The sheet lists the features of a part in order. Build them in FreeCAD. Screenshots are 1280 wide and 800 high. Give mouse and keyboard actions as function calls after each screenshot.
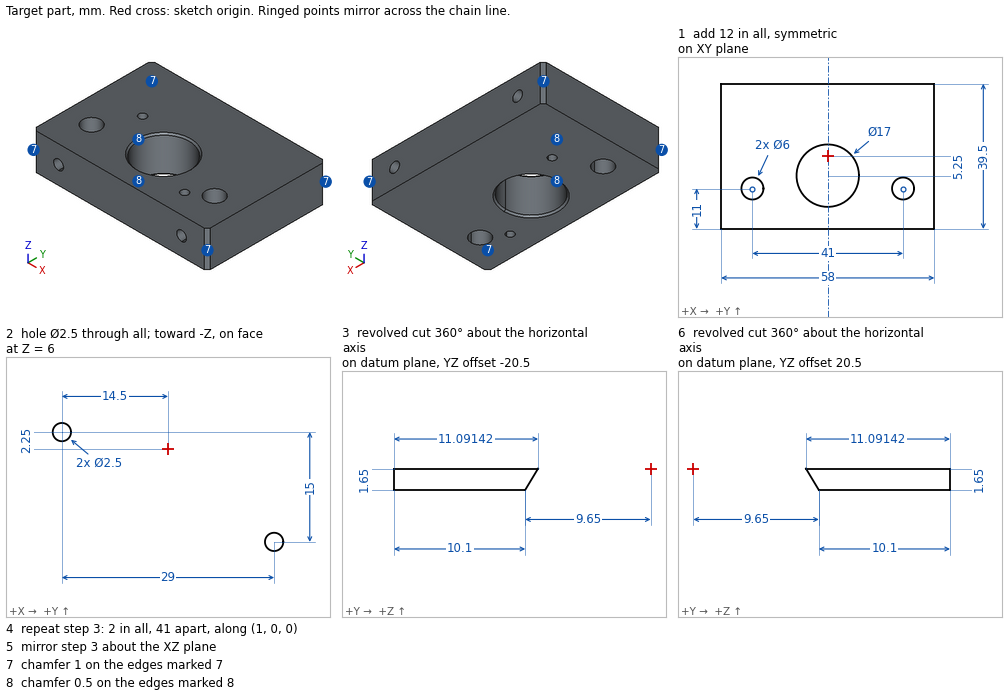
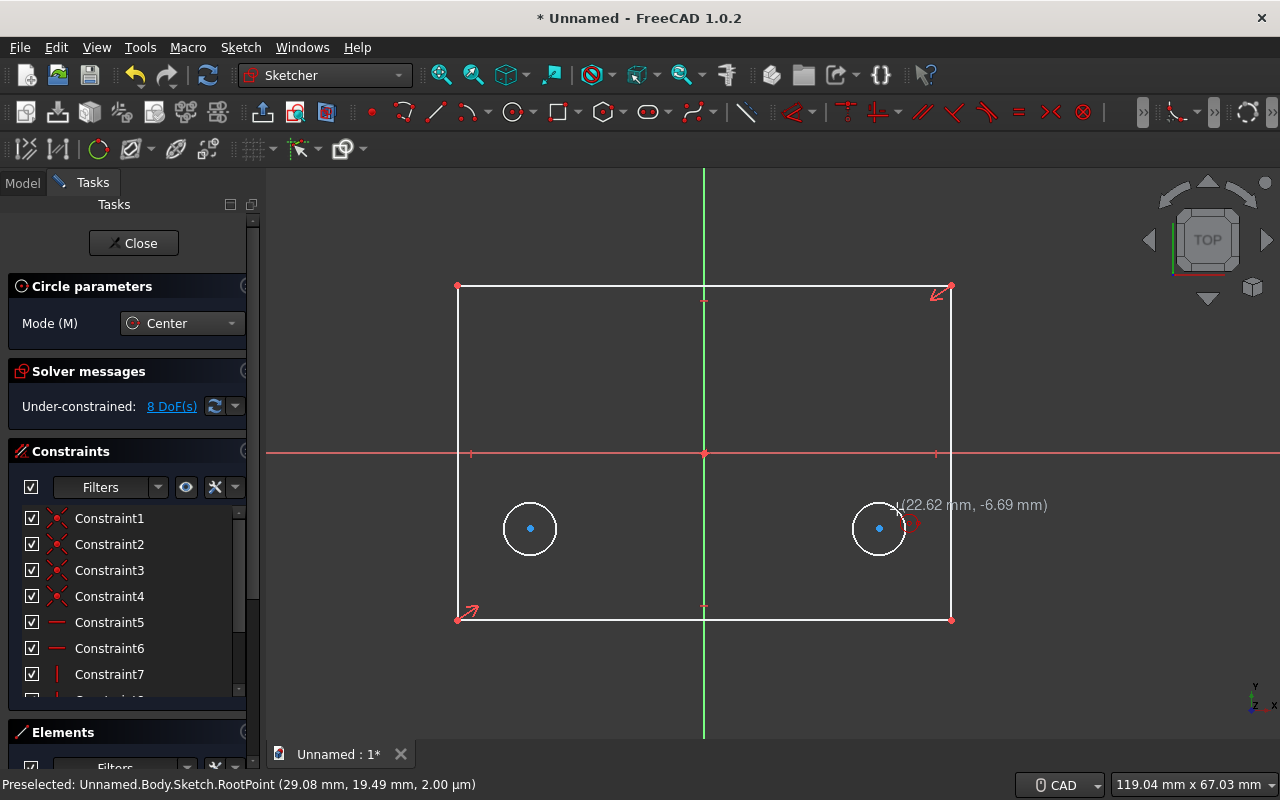
click(704, 498)
click(756, 549)
key(Escape)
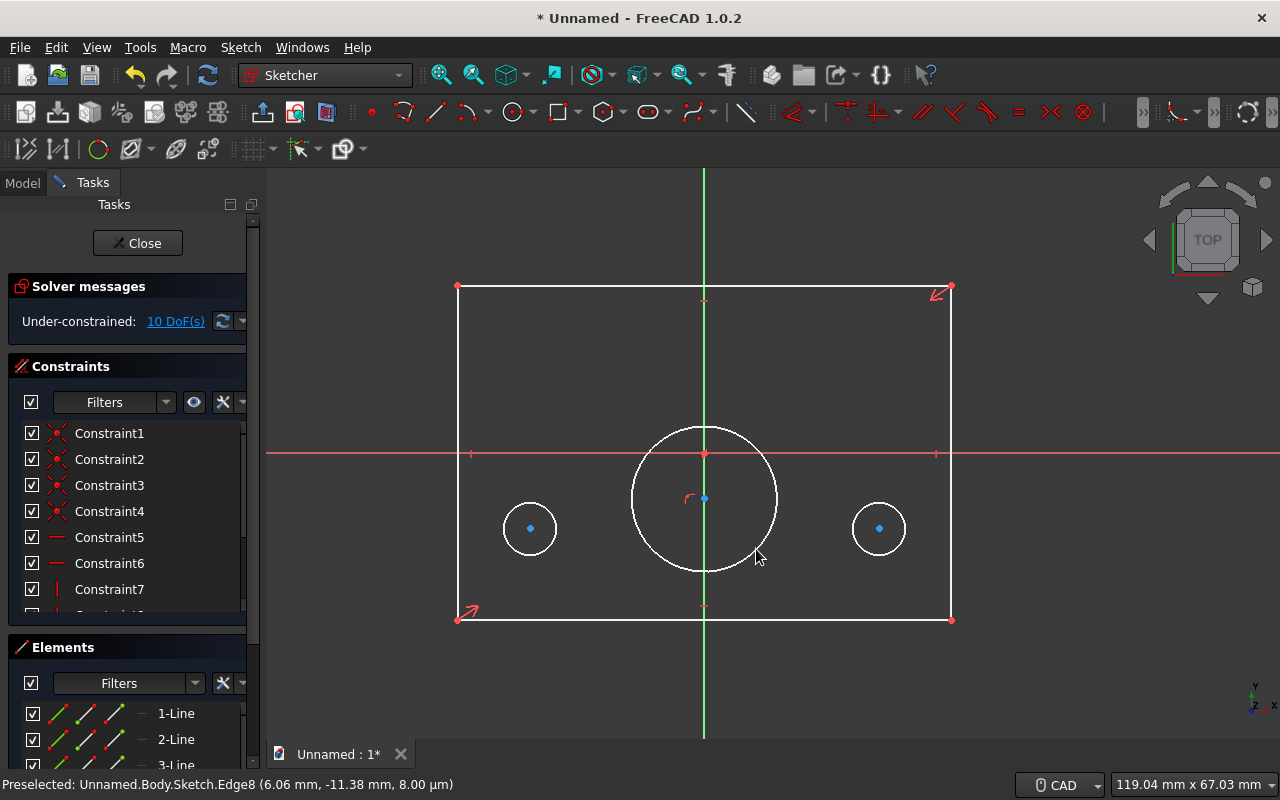
click(548, 510)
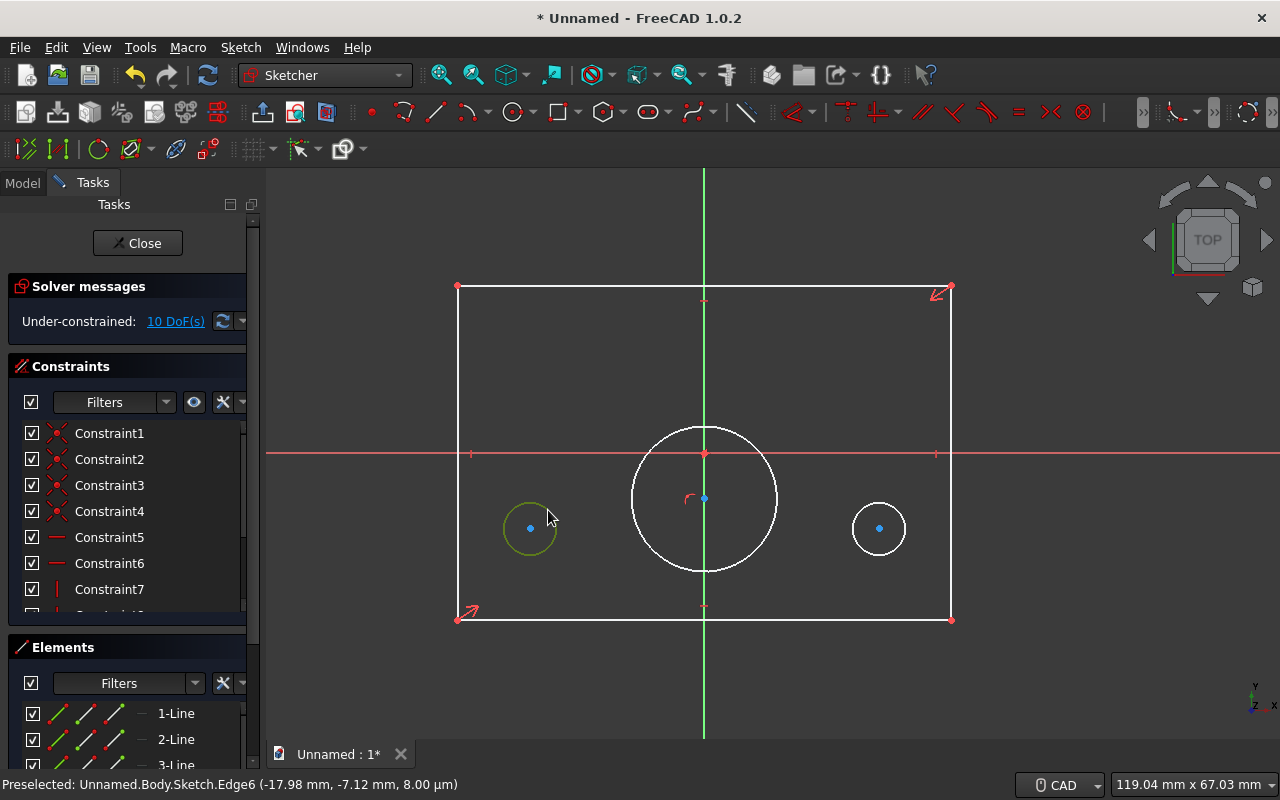
click(897, 510)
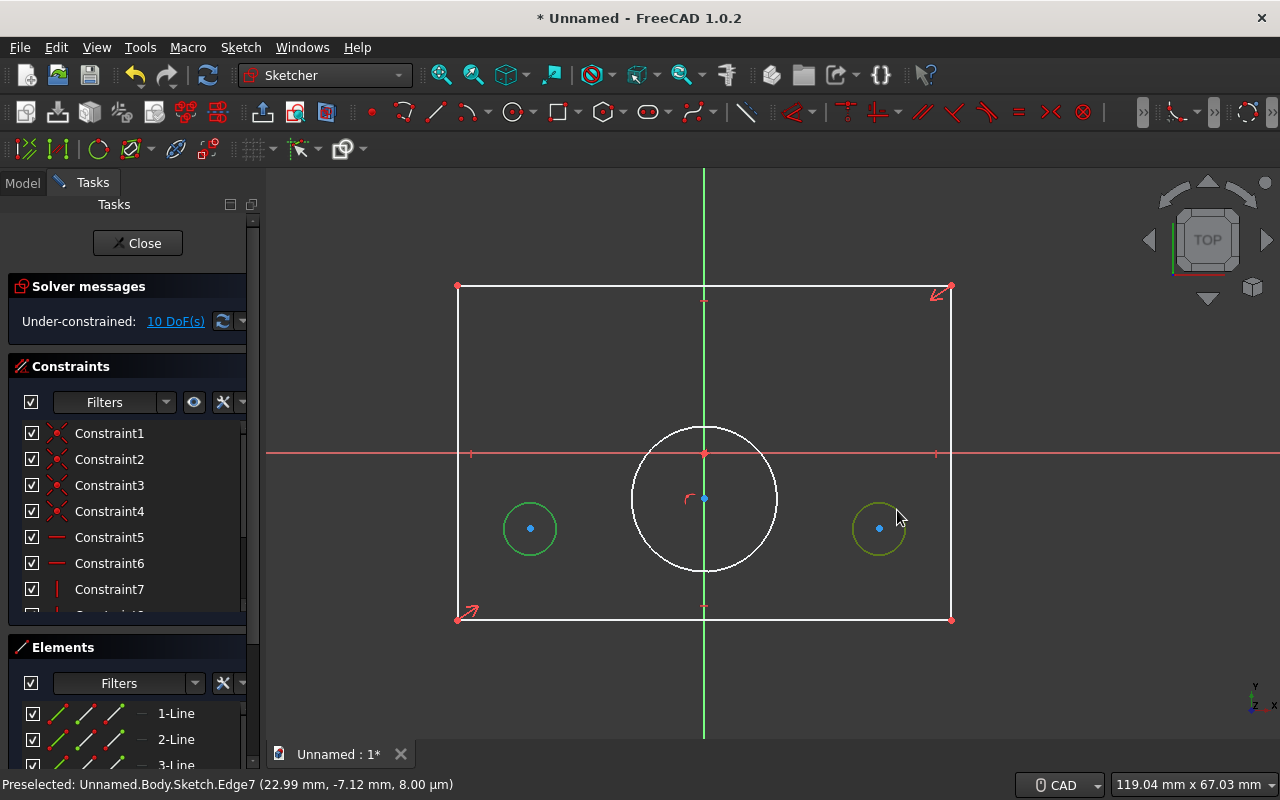
key(e)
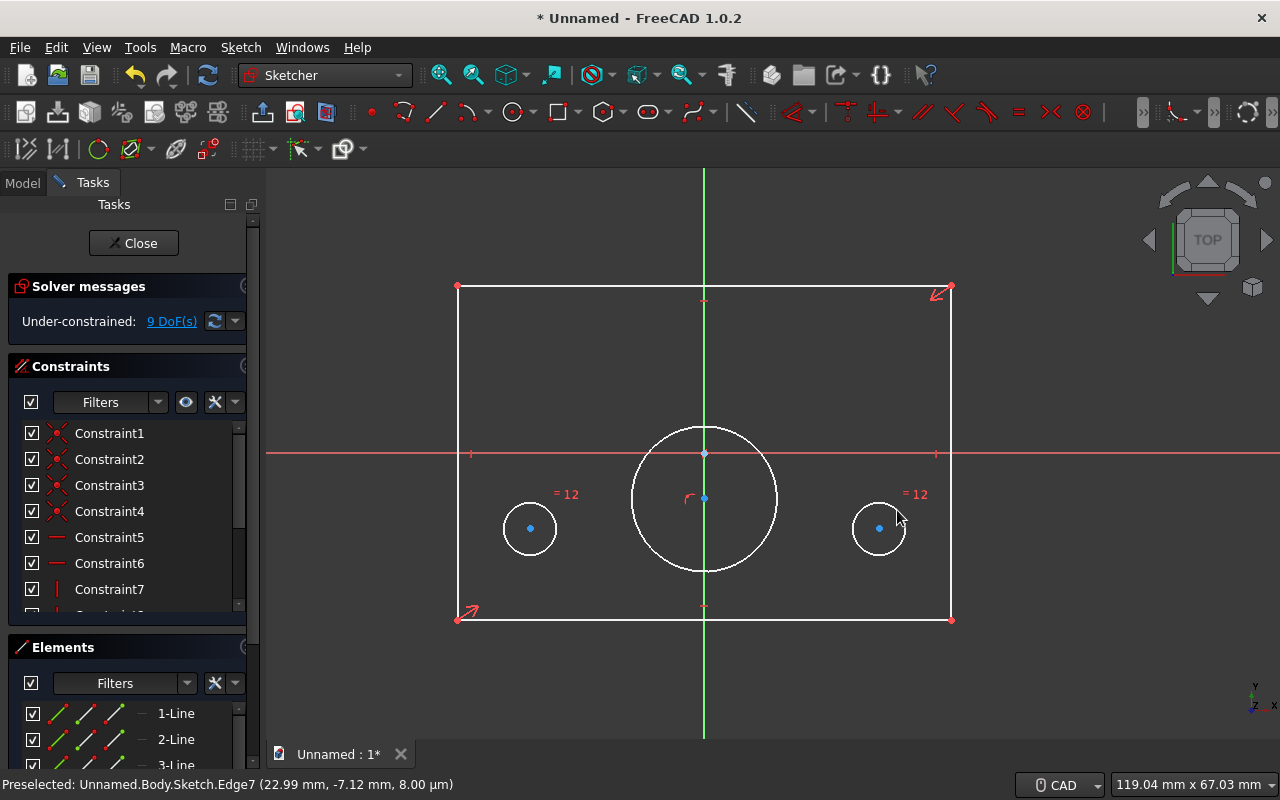
click(530, 529)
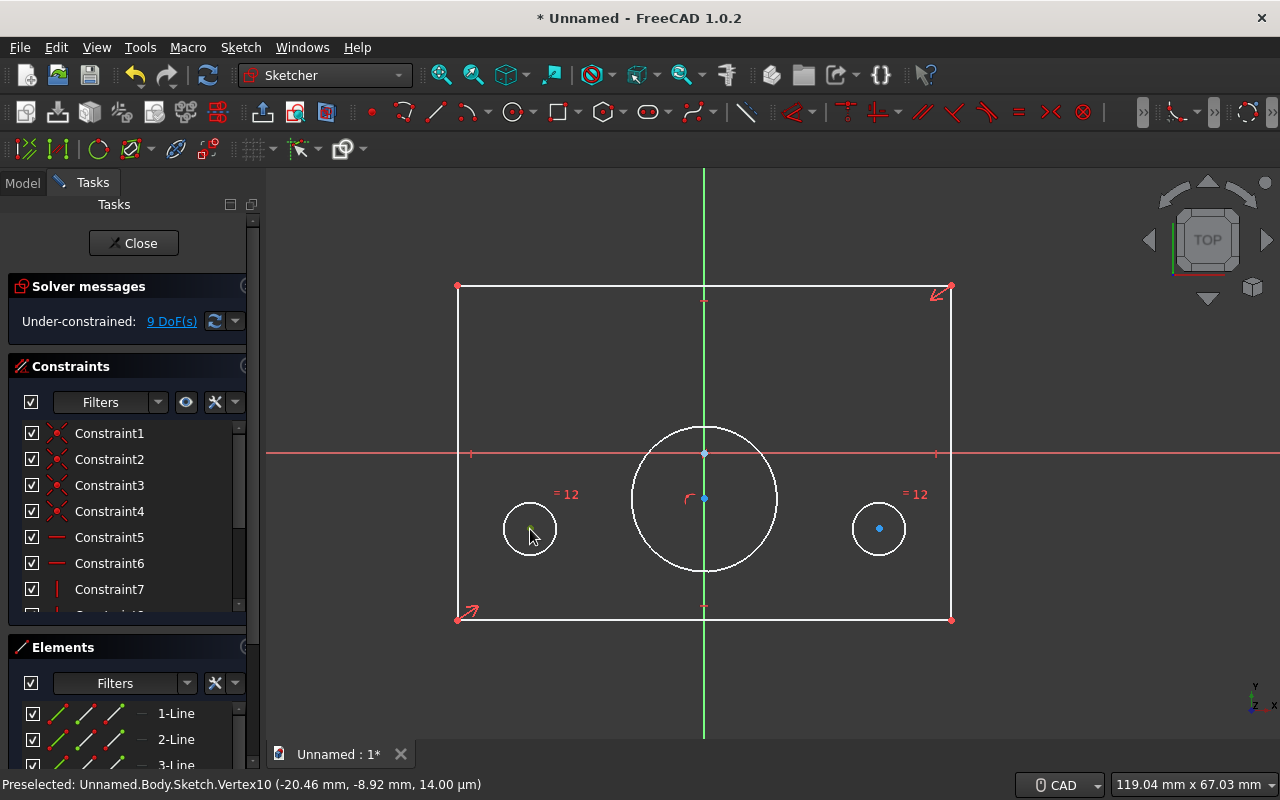
click(879, 529)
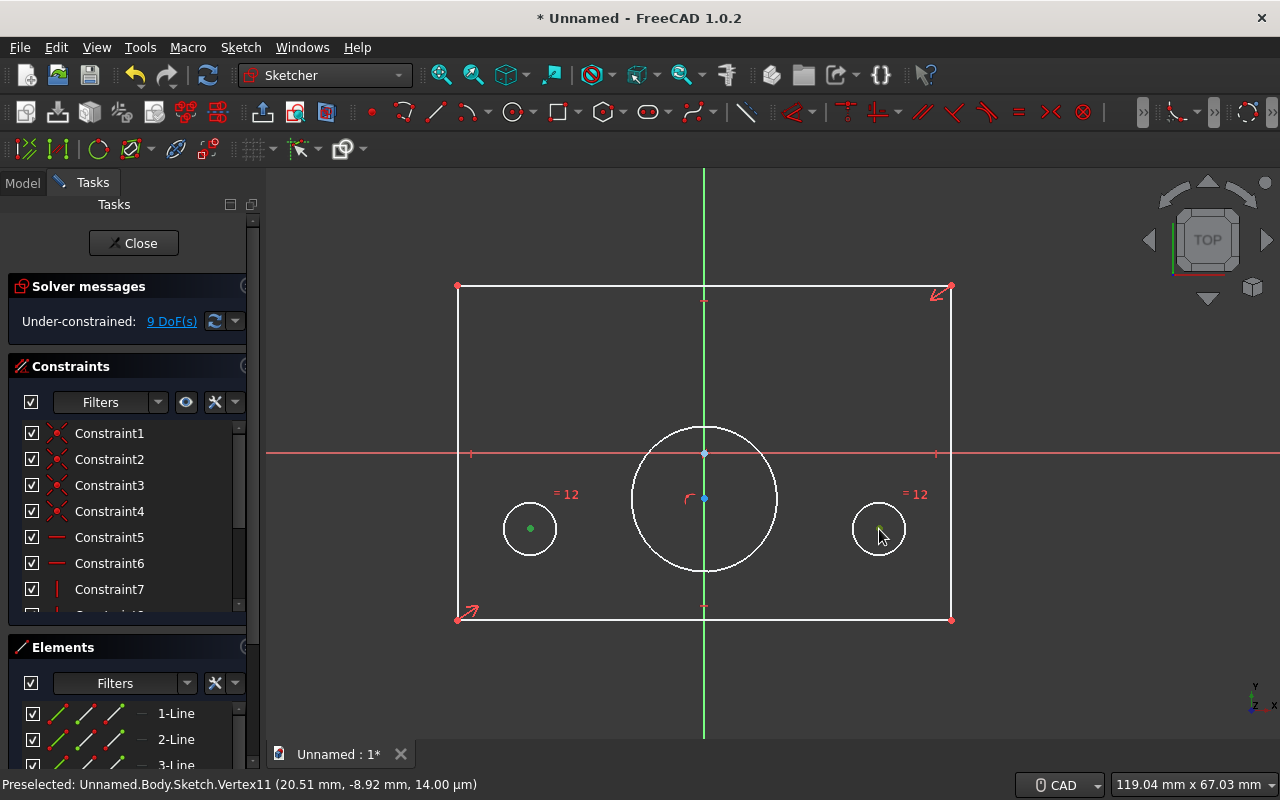
click(704, 674)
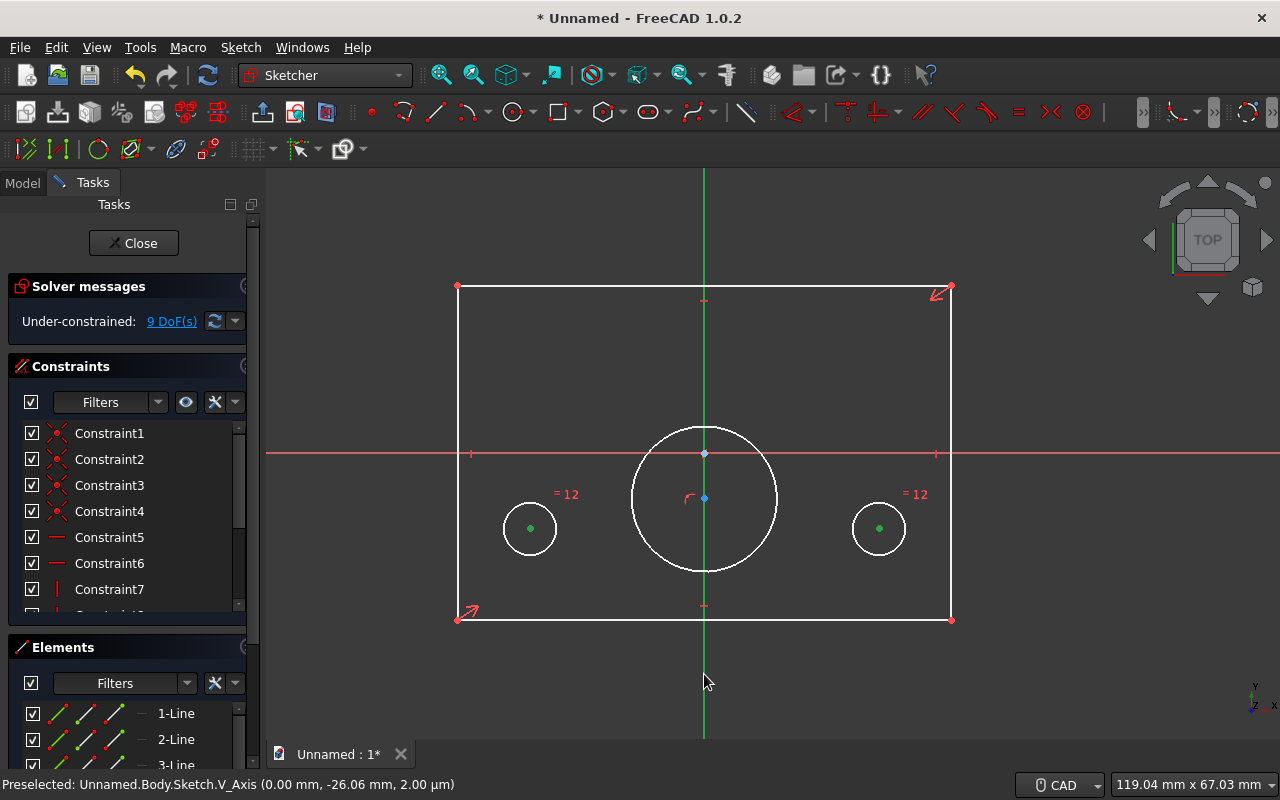
click(1052, 112)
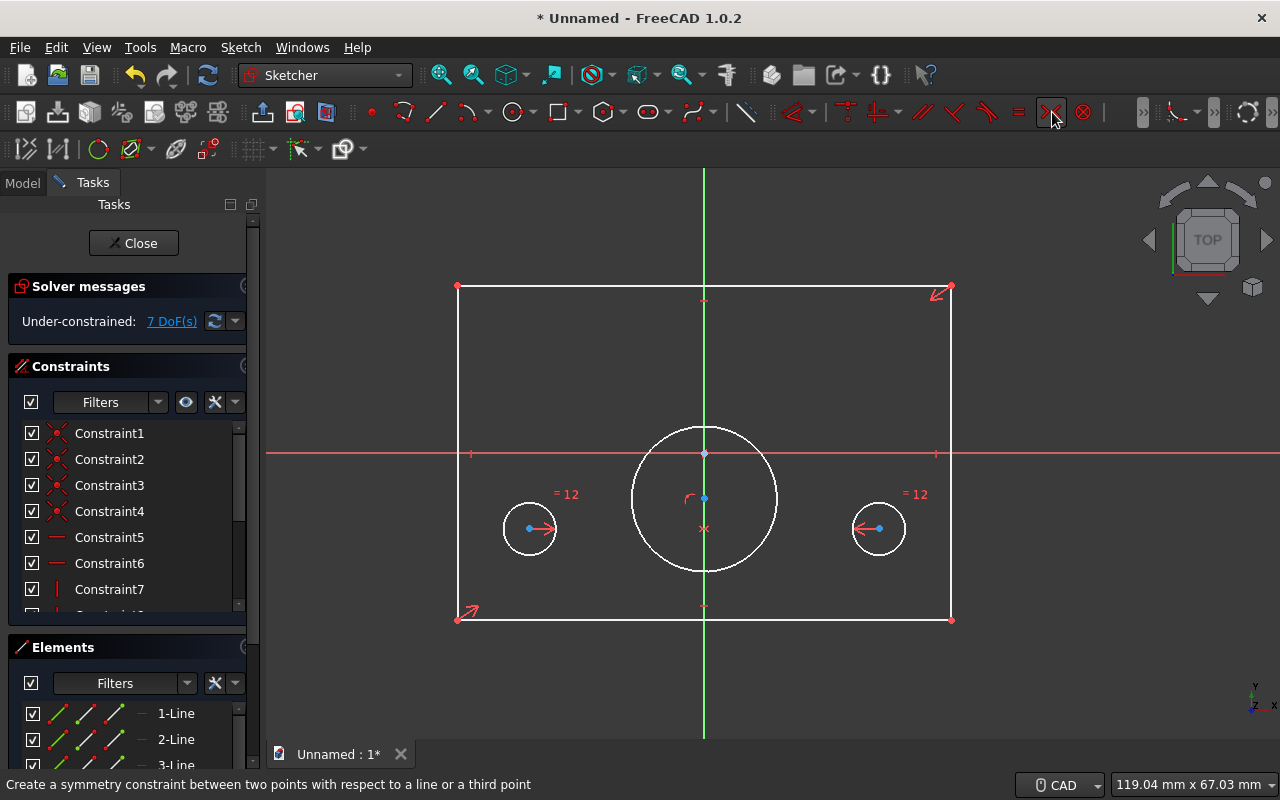
key(d)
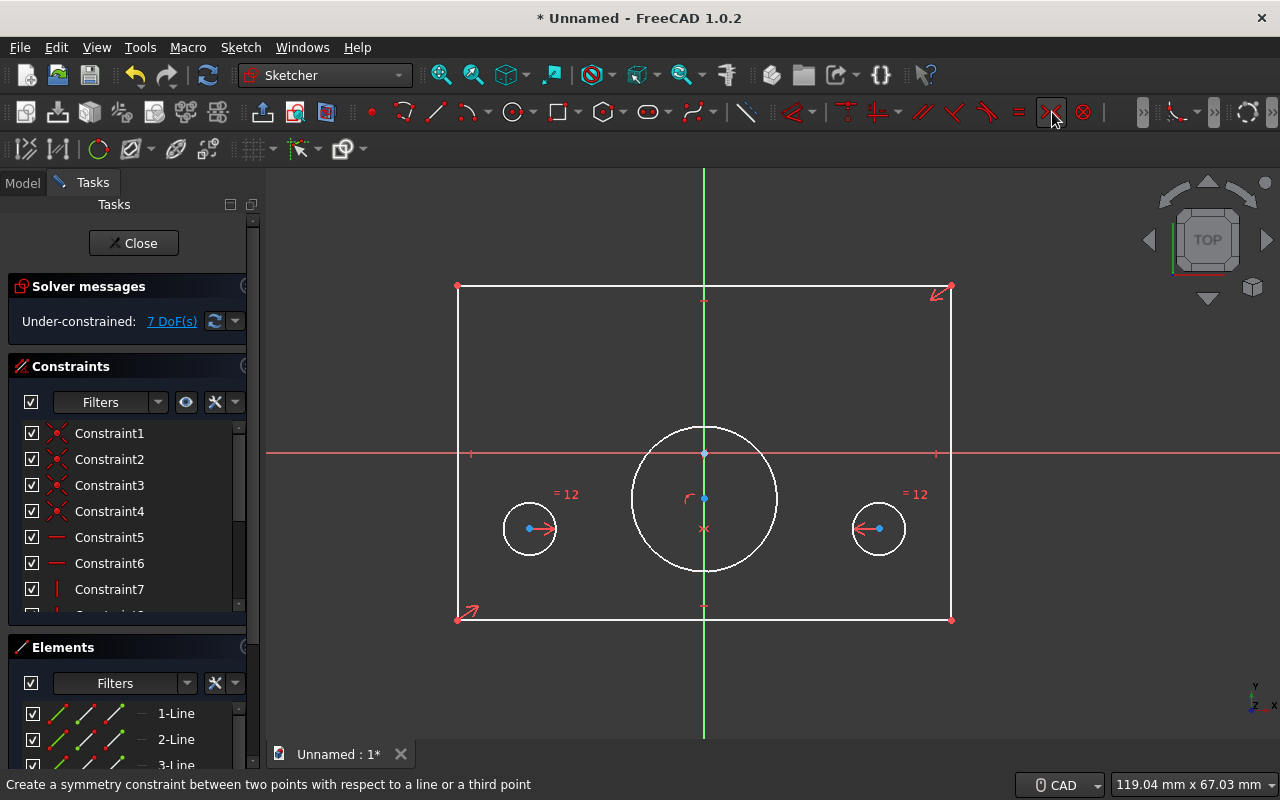
click(548, 510)
click(570, 487)